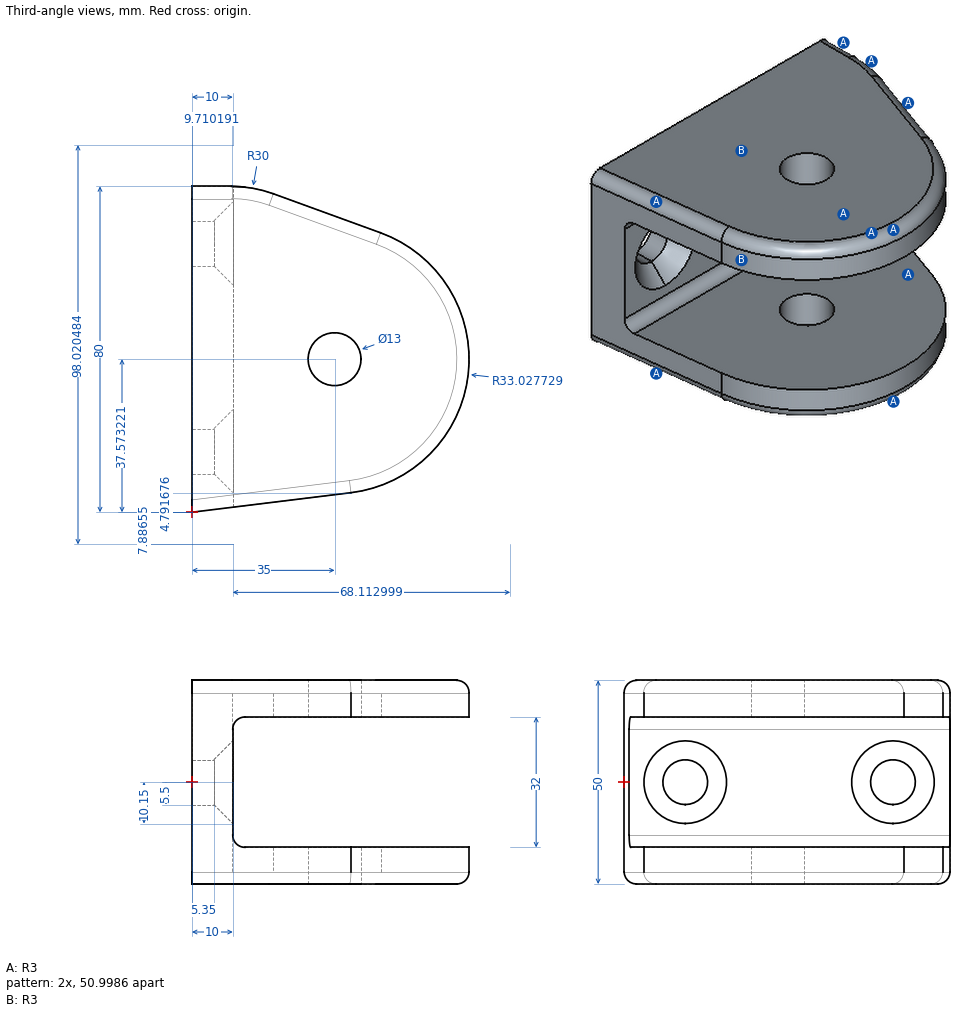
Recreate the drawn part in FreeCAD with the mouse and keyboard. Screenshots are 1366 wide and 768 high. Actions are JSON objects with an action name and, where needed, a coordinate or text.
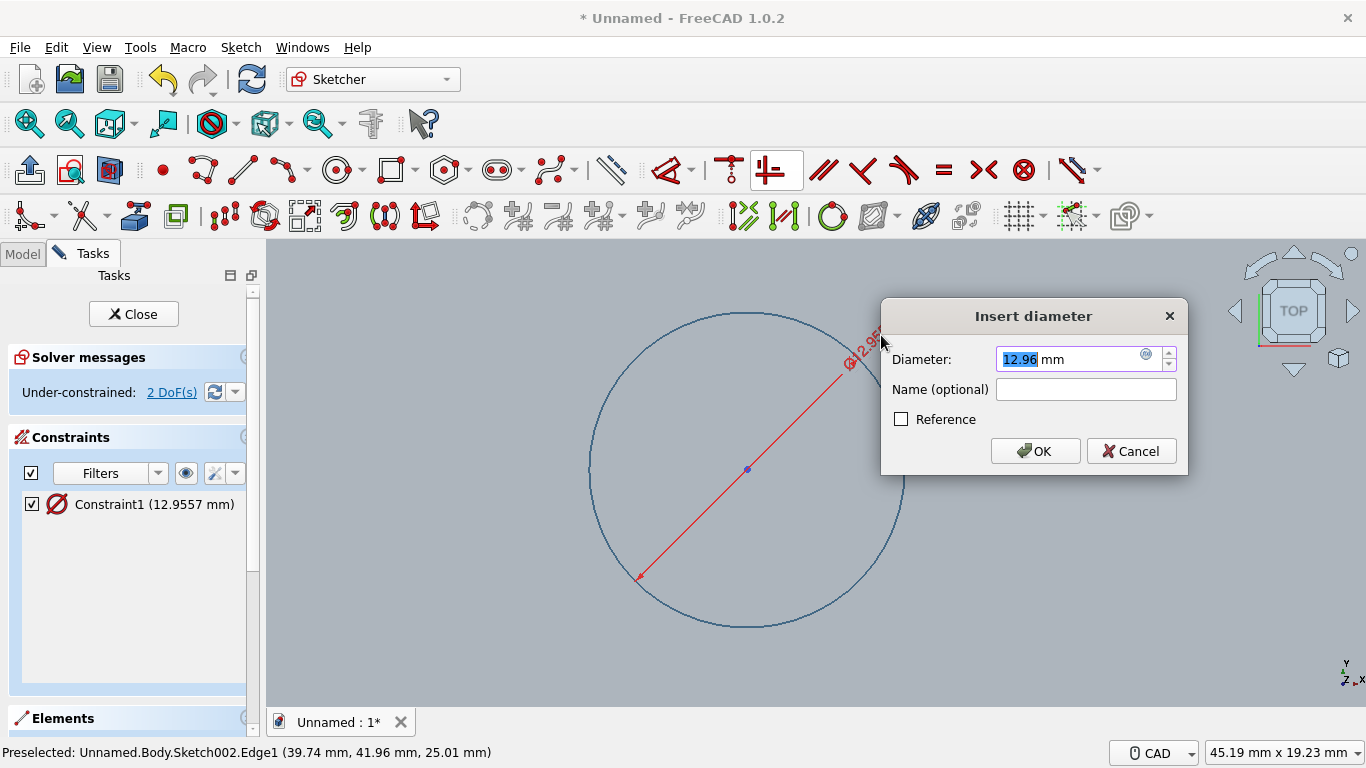
{"action": "type", "text": "13"}
{"action": "key", "text": "Return"}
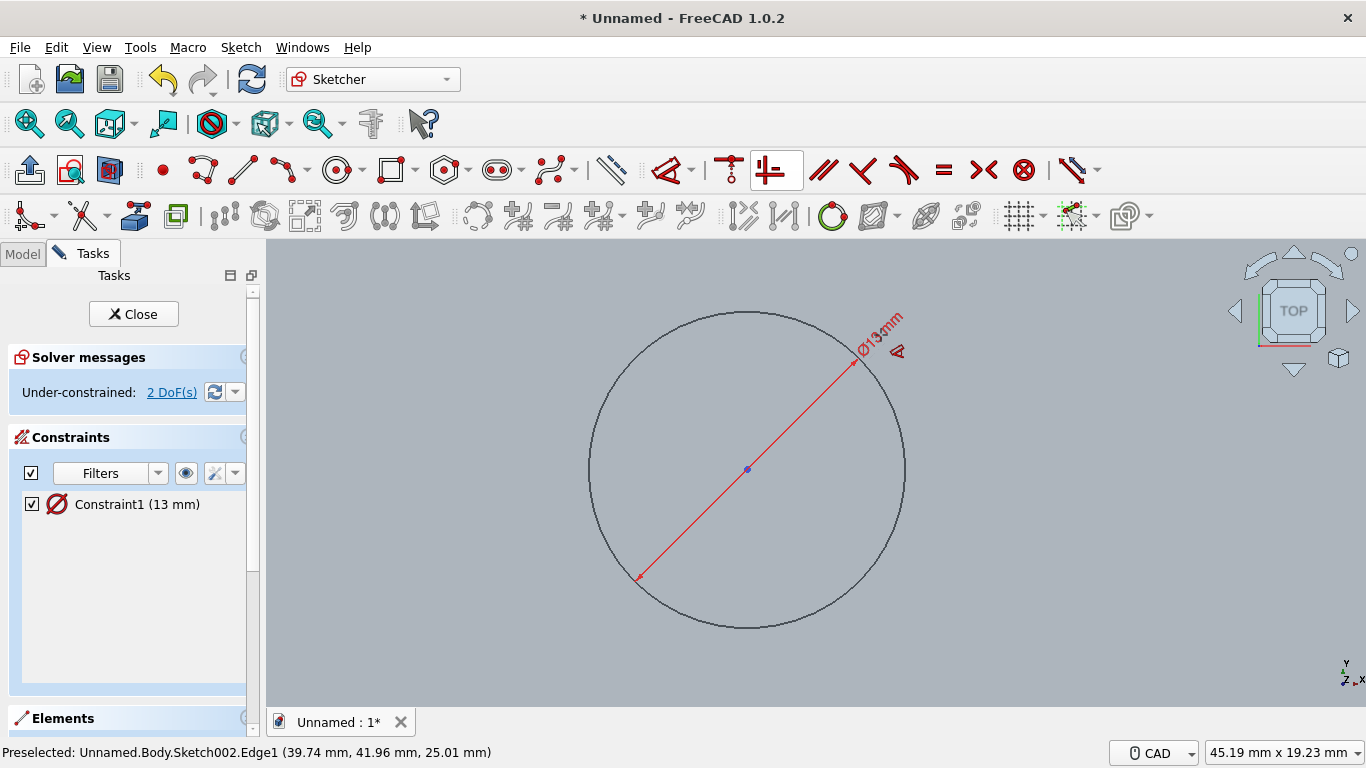
{"action": "left_click", "coordinate": [747, 470]}
{"action": "left_click", "coordinate": [521, 436]}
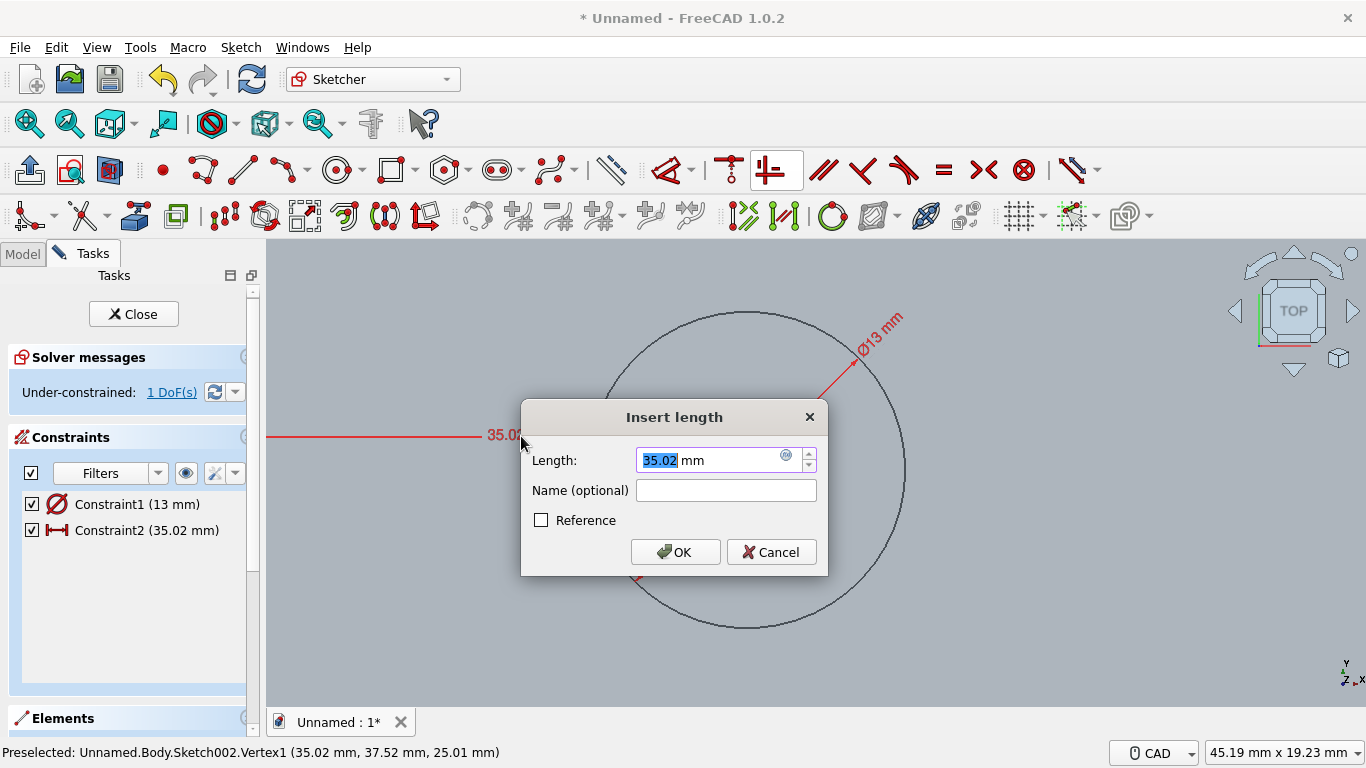
{"action": "type", "text": "35"}
{"action": "key", "text": "Return"}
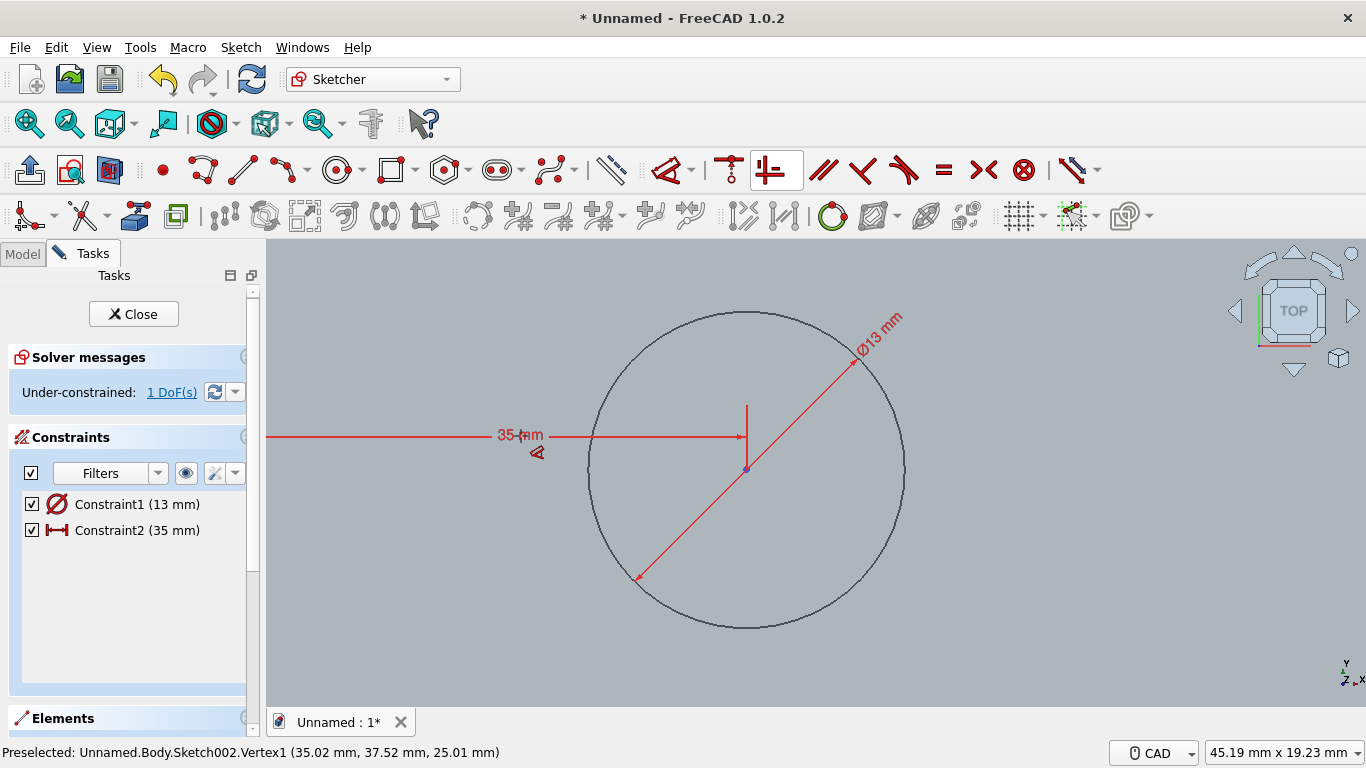
{"action": "left_click", "coordinate": [747, 470]}
{"action": "left_click", "coordinate": [781, 574]}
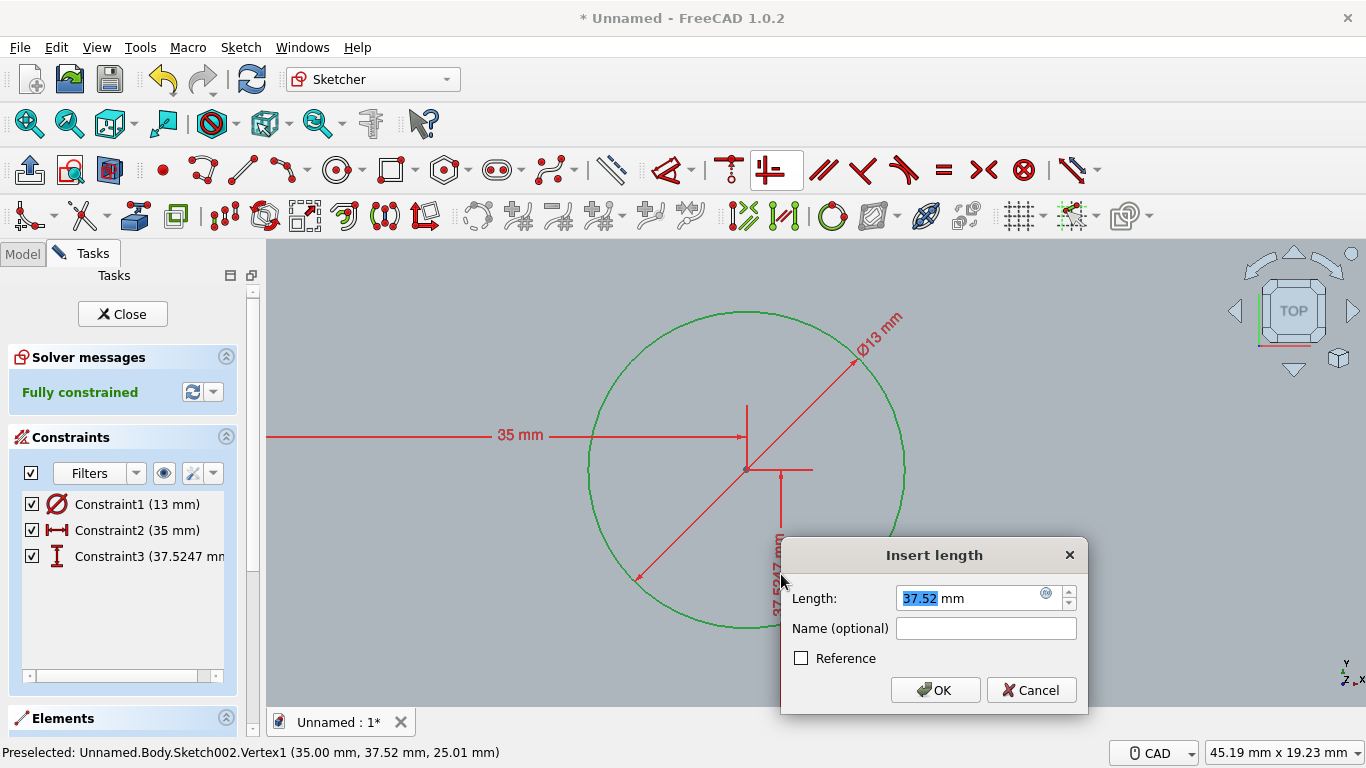
{"action": "type", "text": "37.573221"}
{"action": "key", "text": "Return"}
{"action": "key", "text": "Escape"}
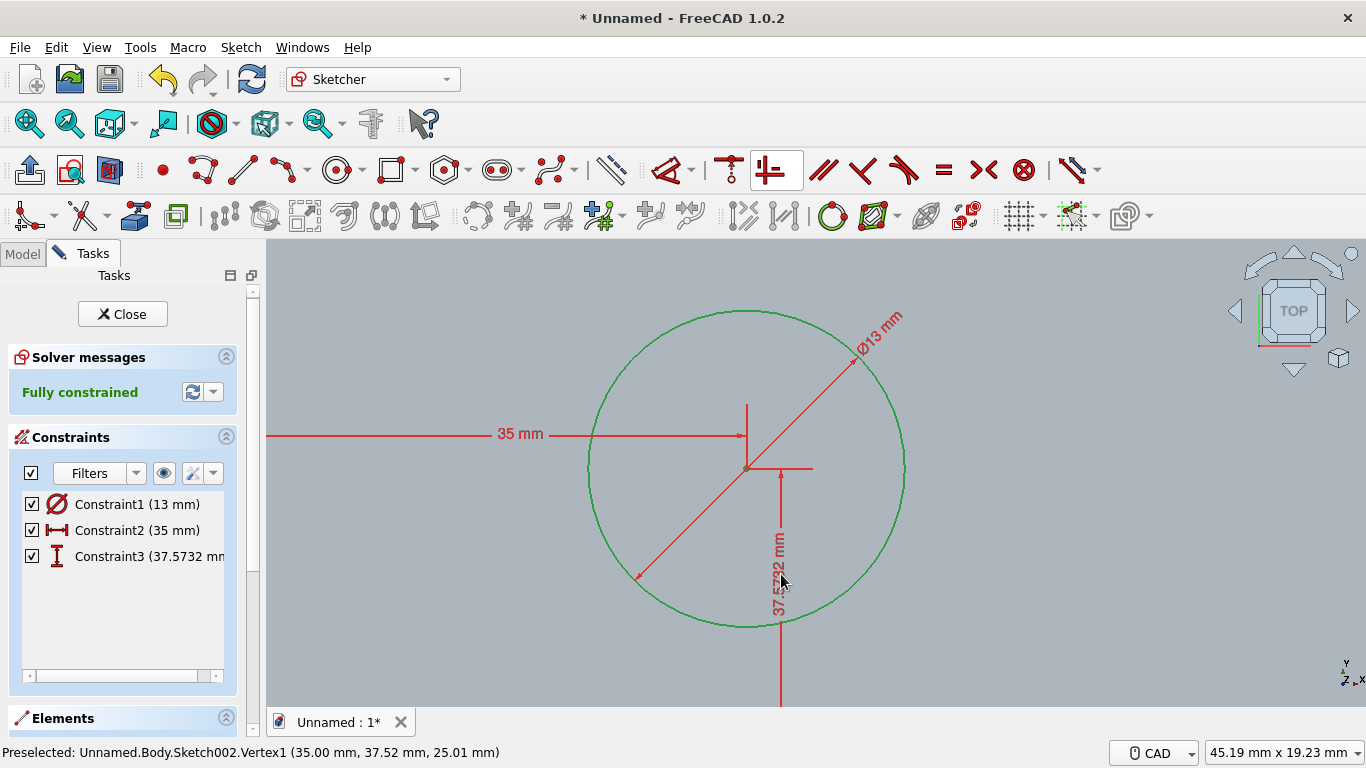
{"action": "left_click", "coordinate": [123, 314]}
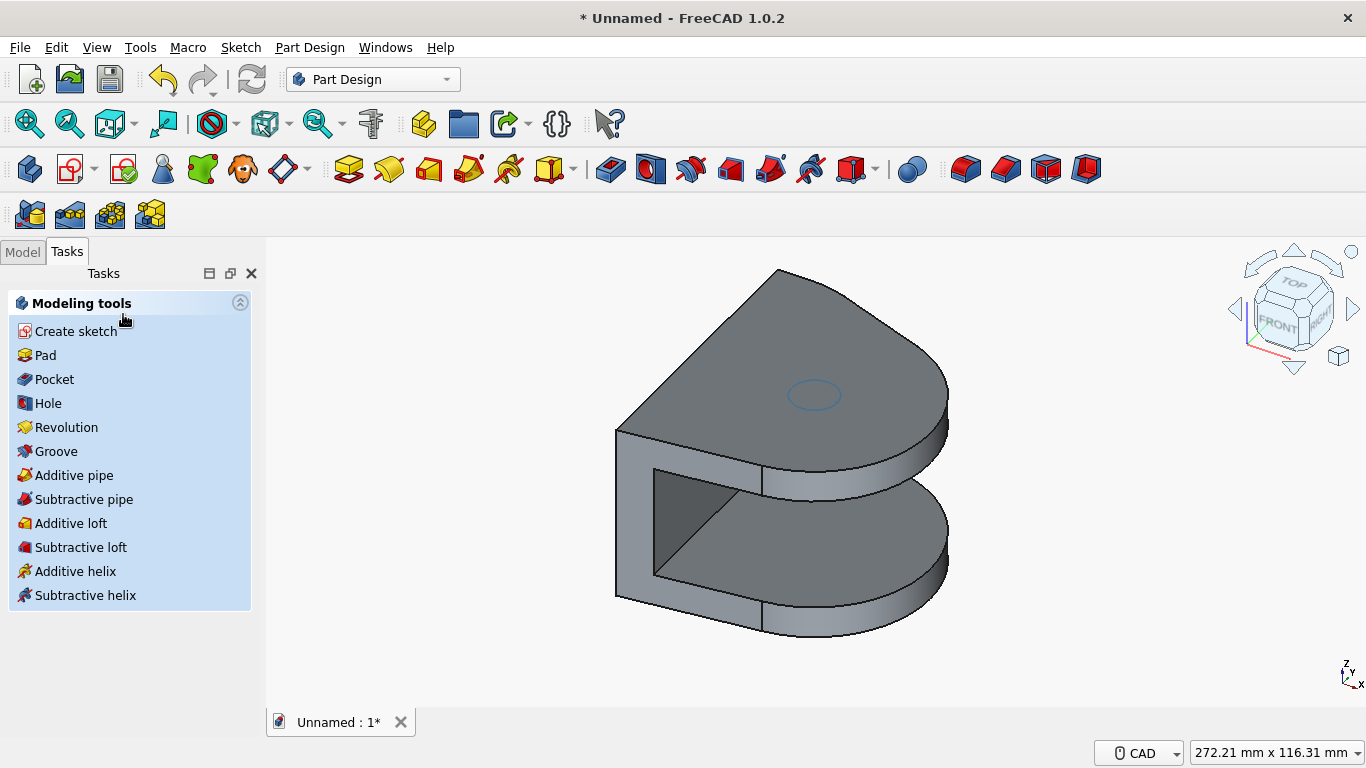
{"action": "left_click", "coordinate": [612, 170]}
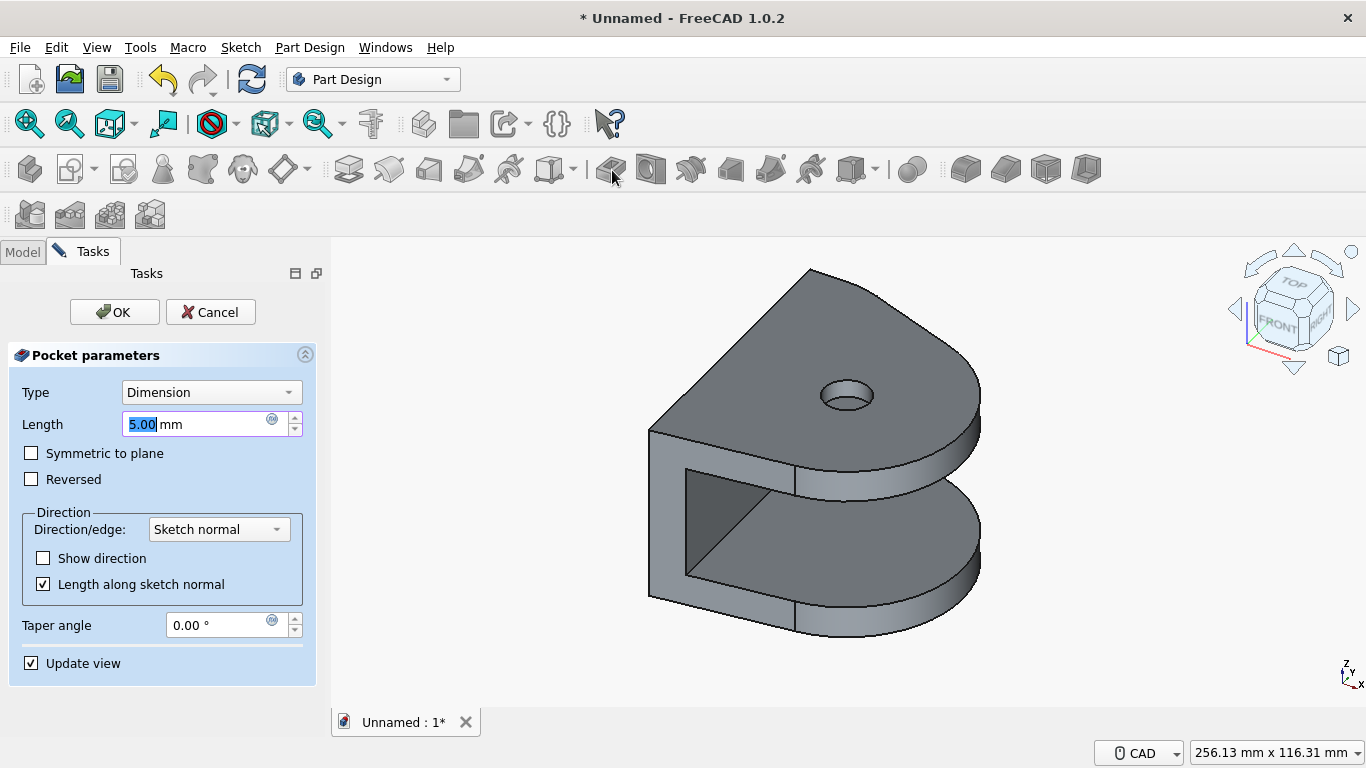
{"action": "left_click", "coordinate": [212, 392]}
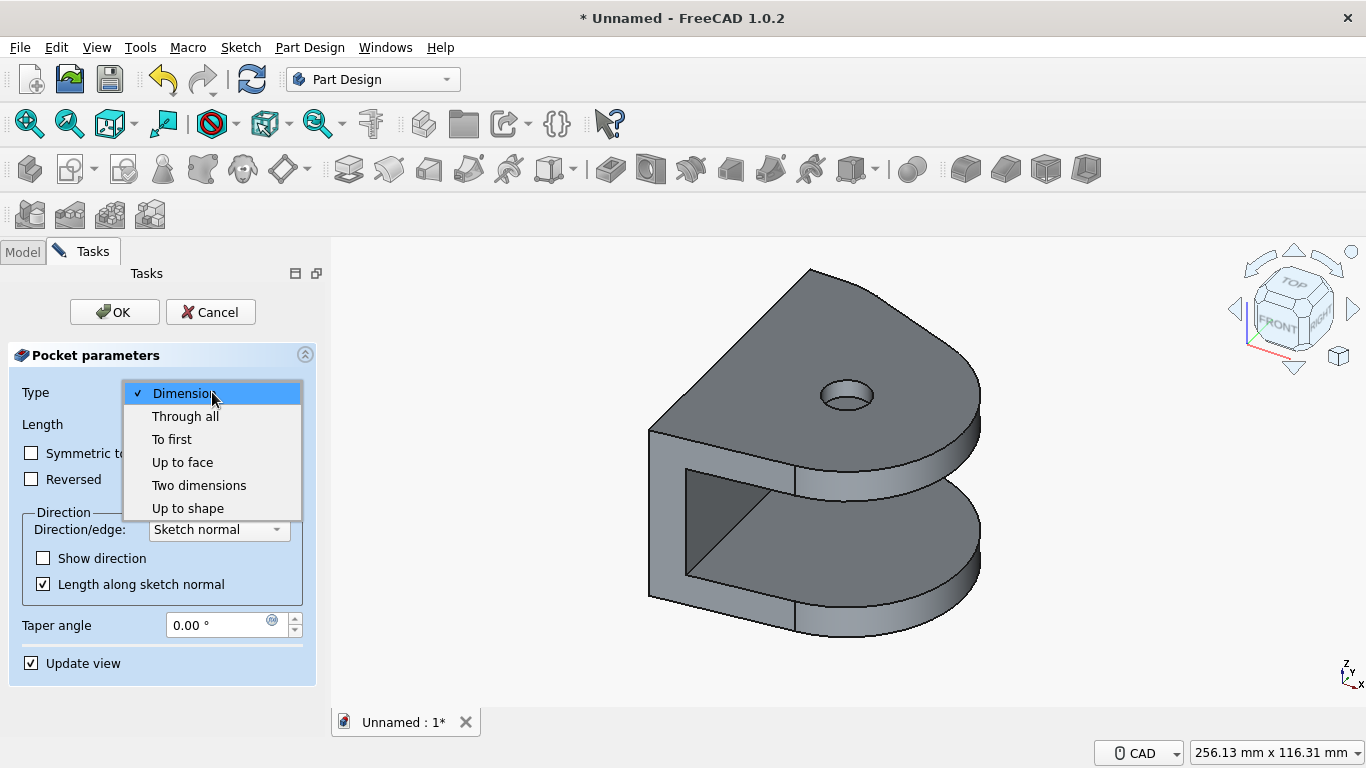
{"action": "left_click", "coordinate": [212, 416]}